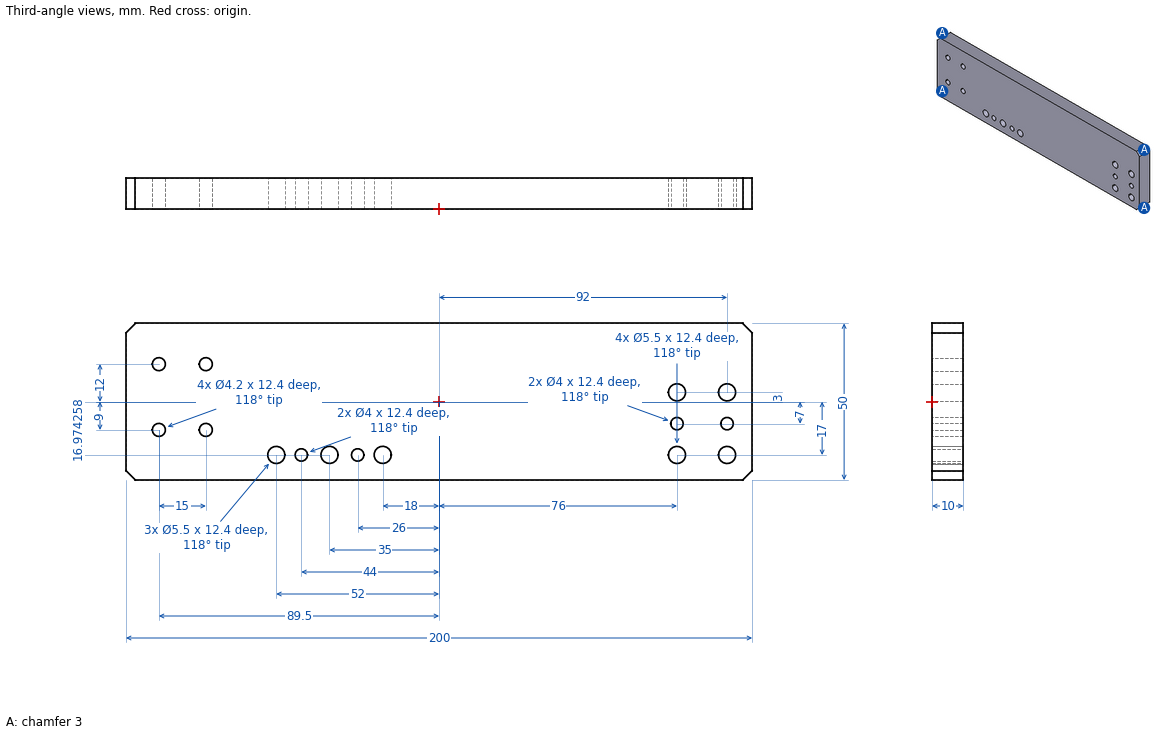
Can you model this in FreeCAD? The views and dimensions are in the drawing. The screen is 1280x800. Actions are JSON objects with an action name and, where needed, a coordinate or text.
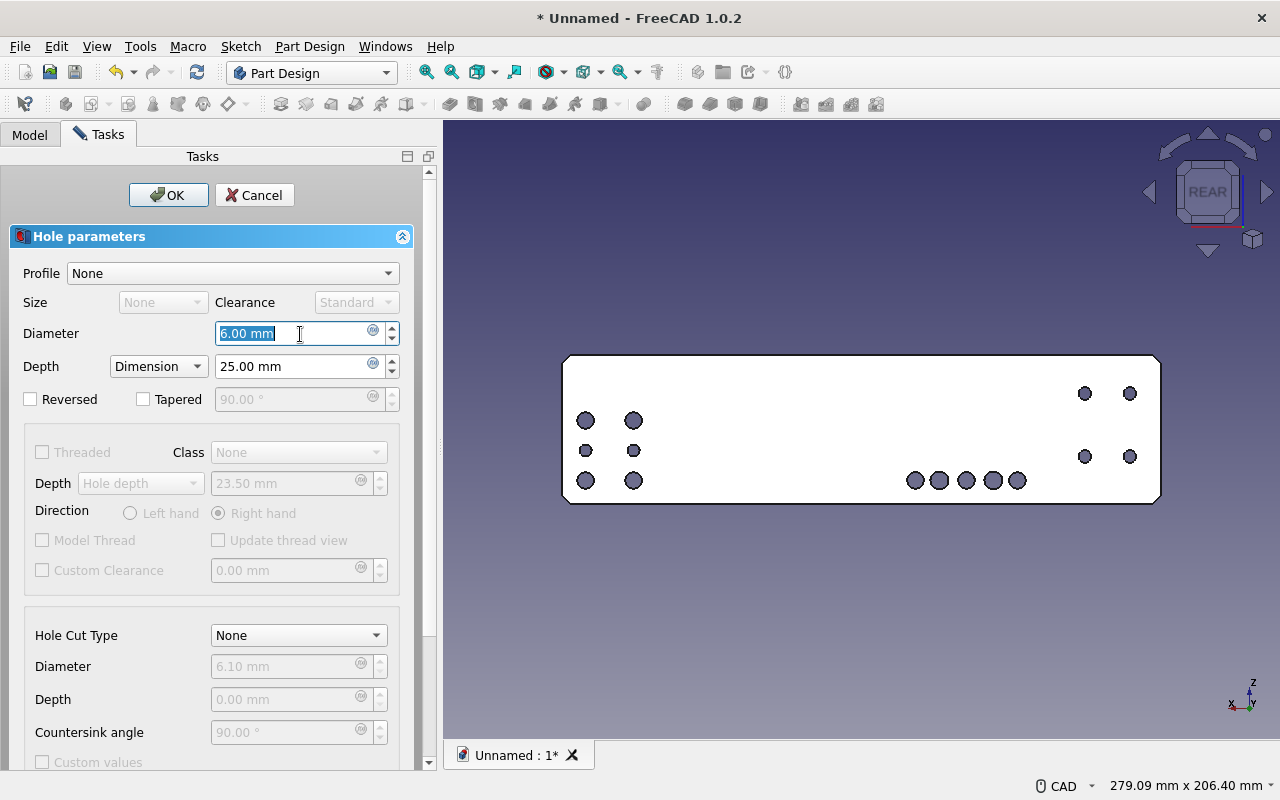
{"action": "type", "text": "4"}
{"action": "key", "text": "Tab"}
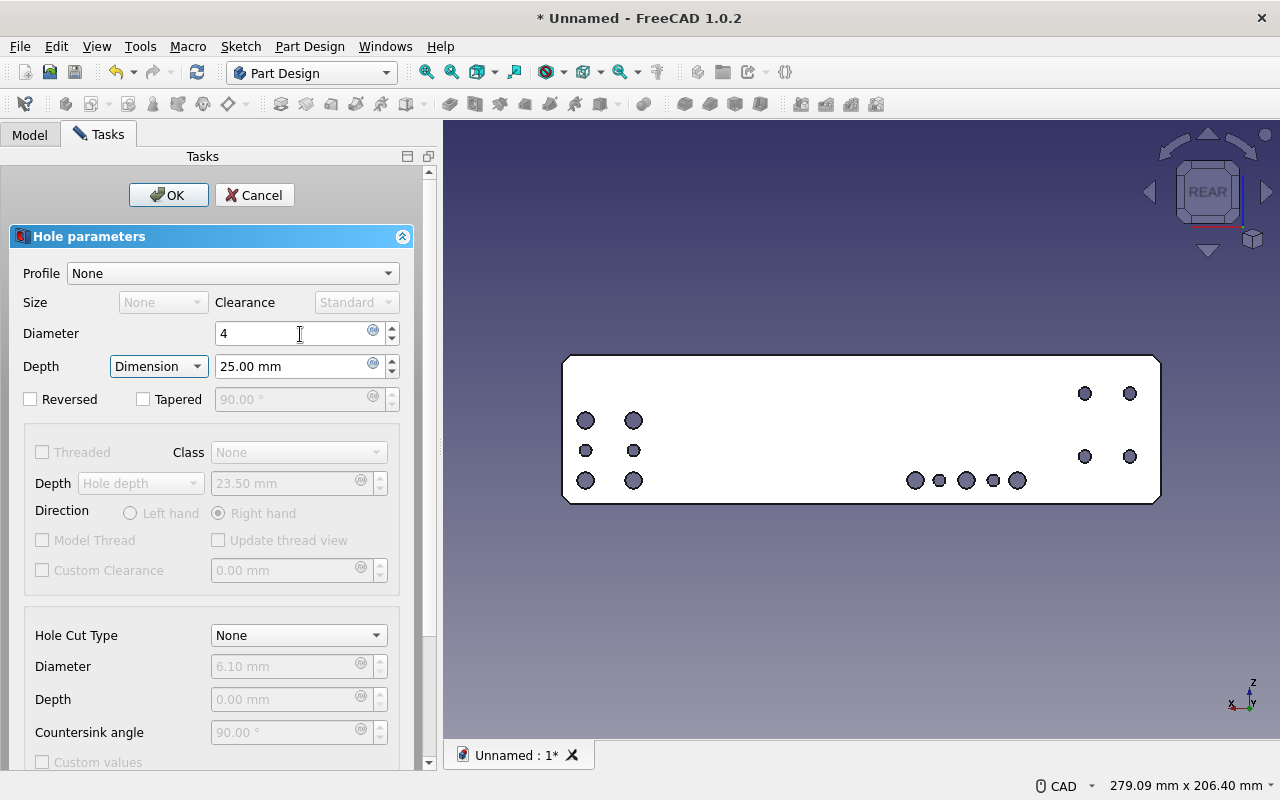
{"action": "triple_click", "coordinate": [300, 366]}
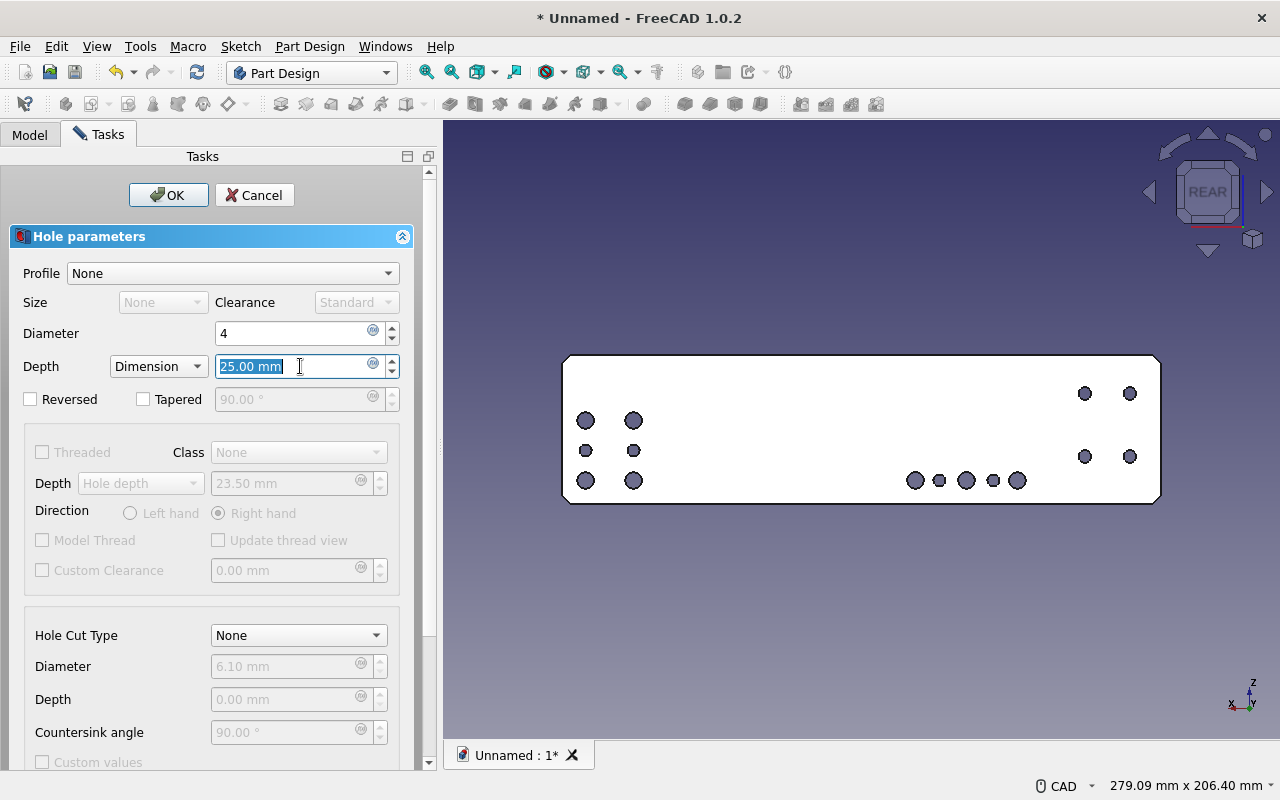
{"action": "type", "text": "12.4"}
{"action": "key", "text": "Tab"}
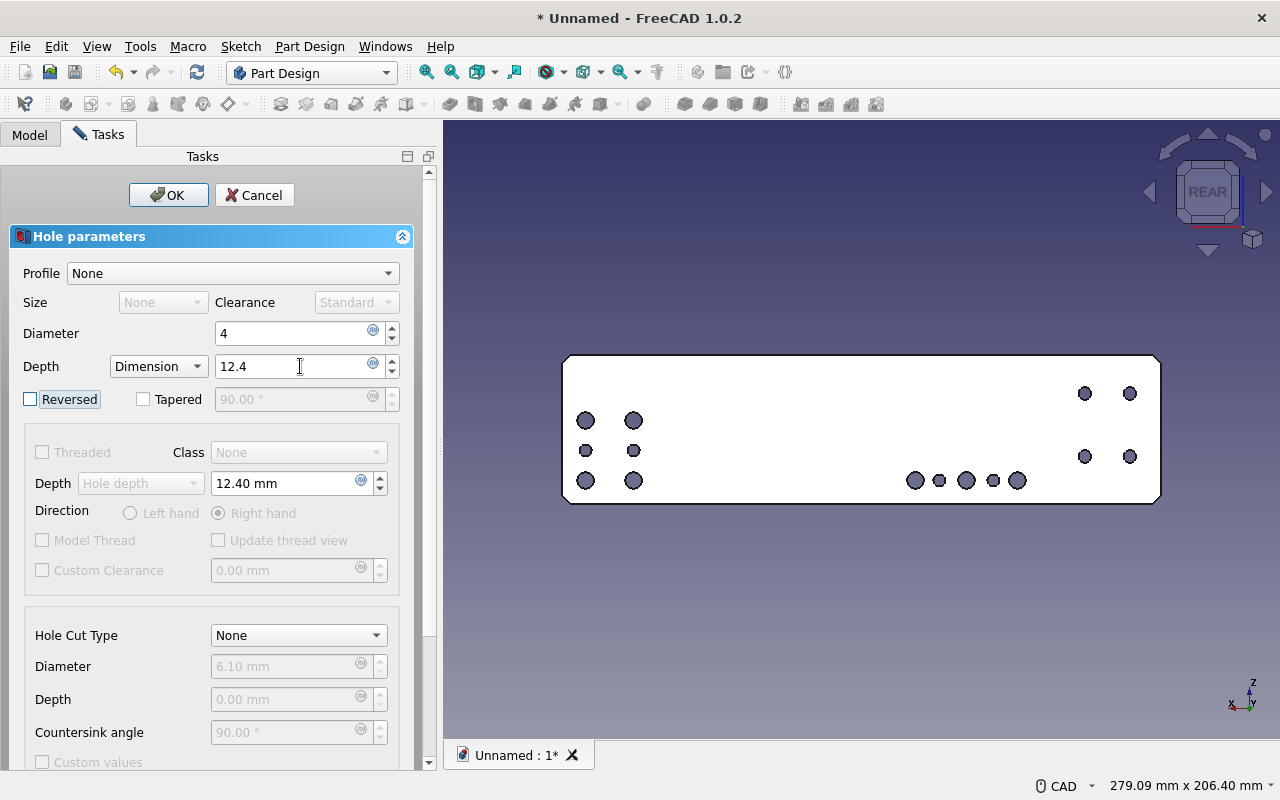
{"action": "left_click", "coordinate": [169, 195]}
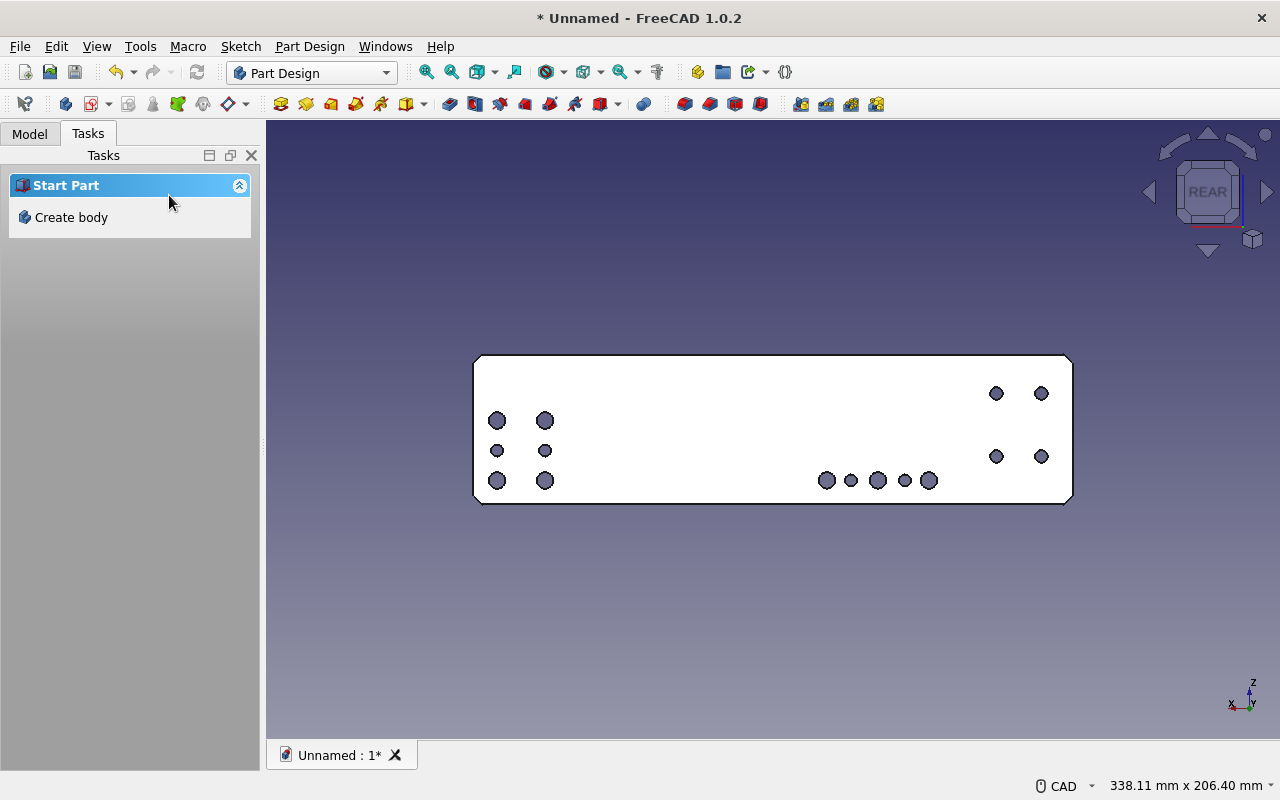
{"action": "key", "text": "0"}